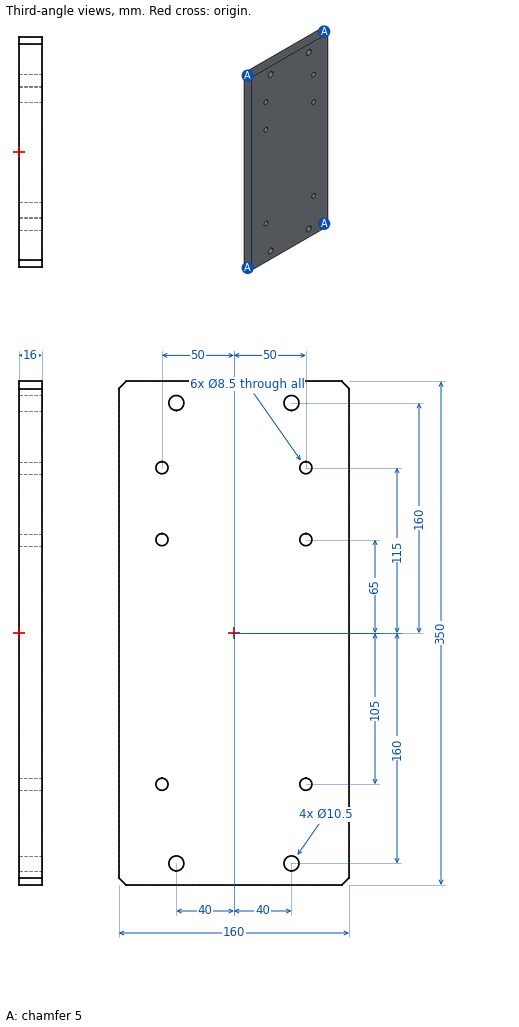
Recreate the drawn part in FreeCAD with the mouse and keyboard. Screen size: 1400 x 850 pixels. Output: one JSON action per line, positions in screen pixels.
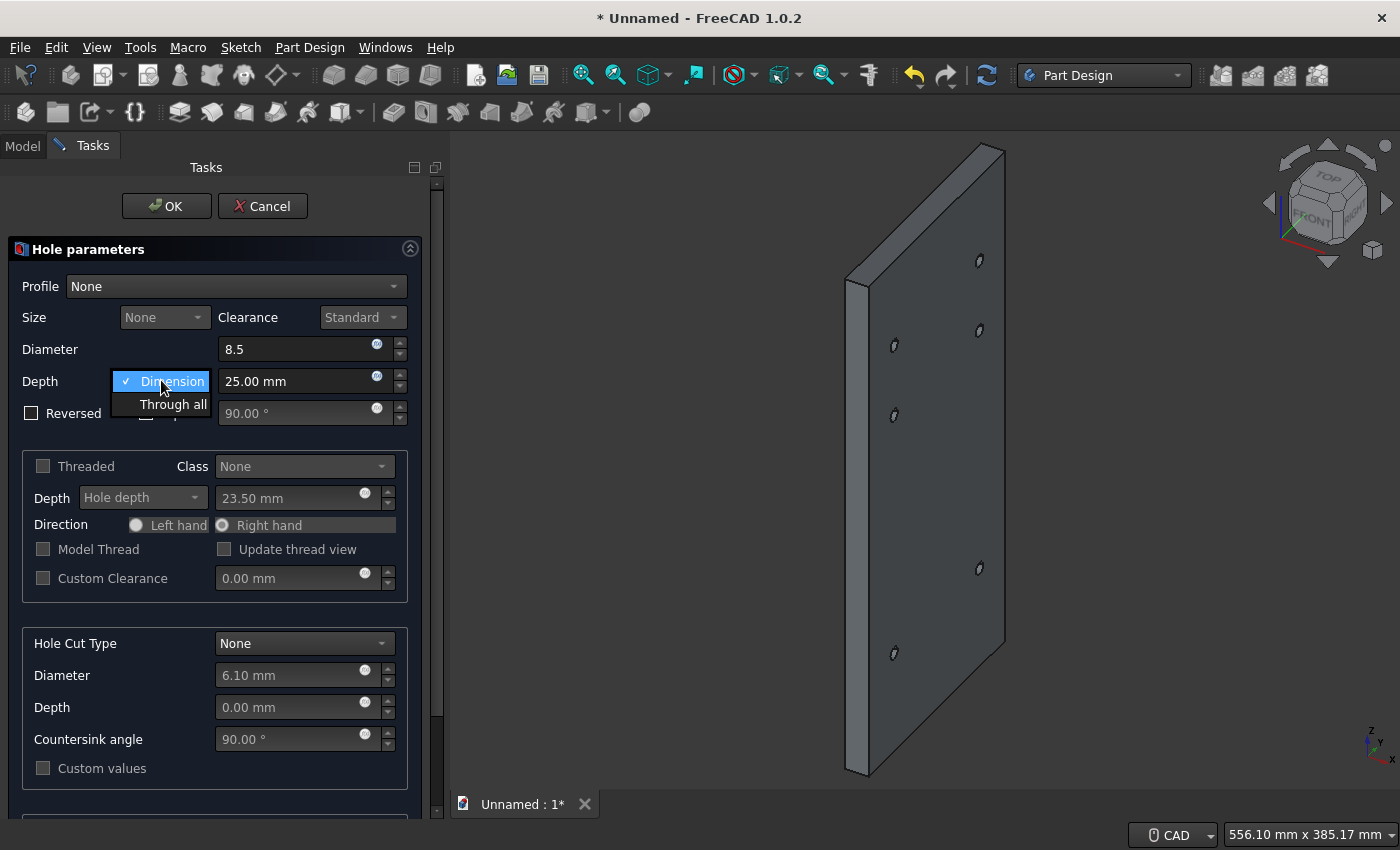
{"action": "left_click", "coordinate": [160, 404]}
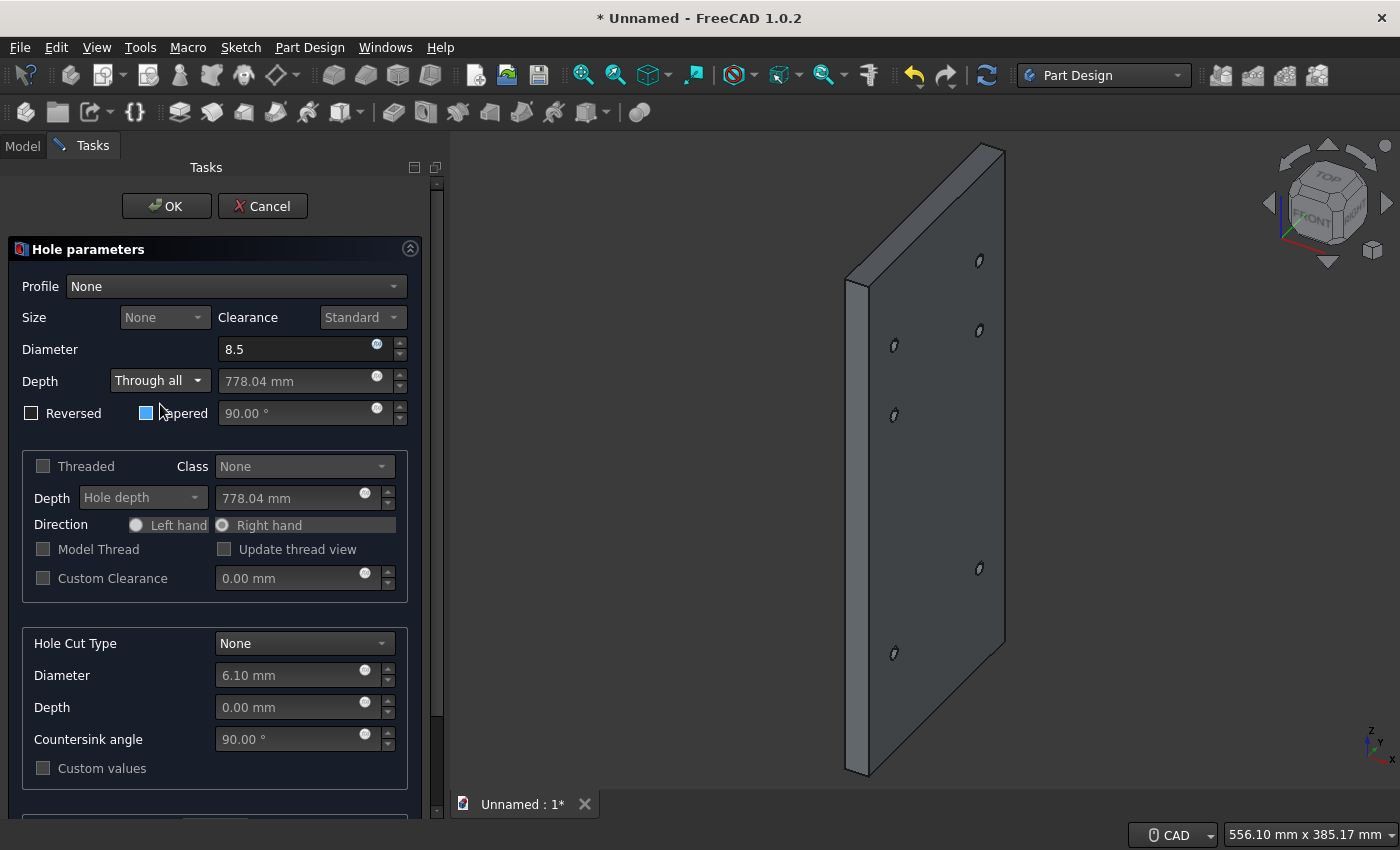
{"action": "left_click", "coordinate": [167, 206]}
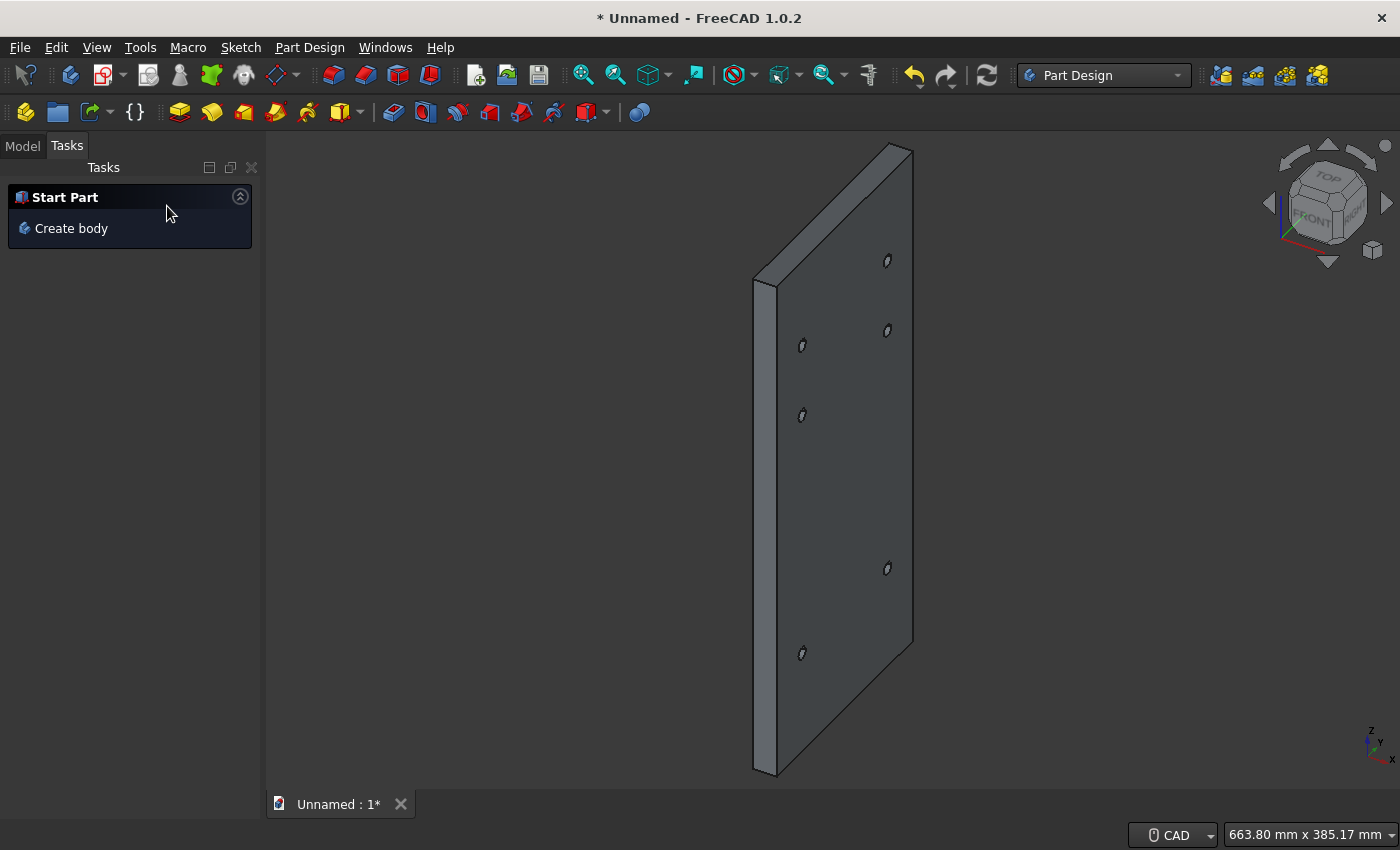
{"action": "key", "text": "6"}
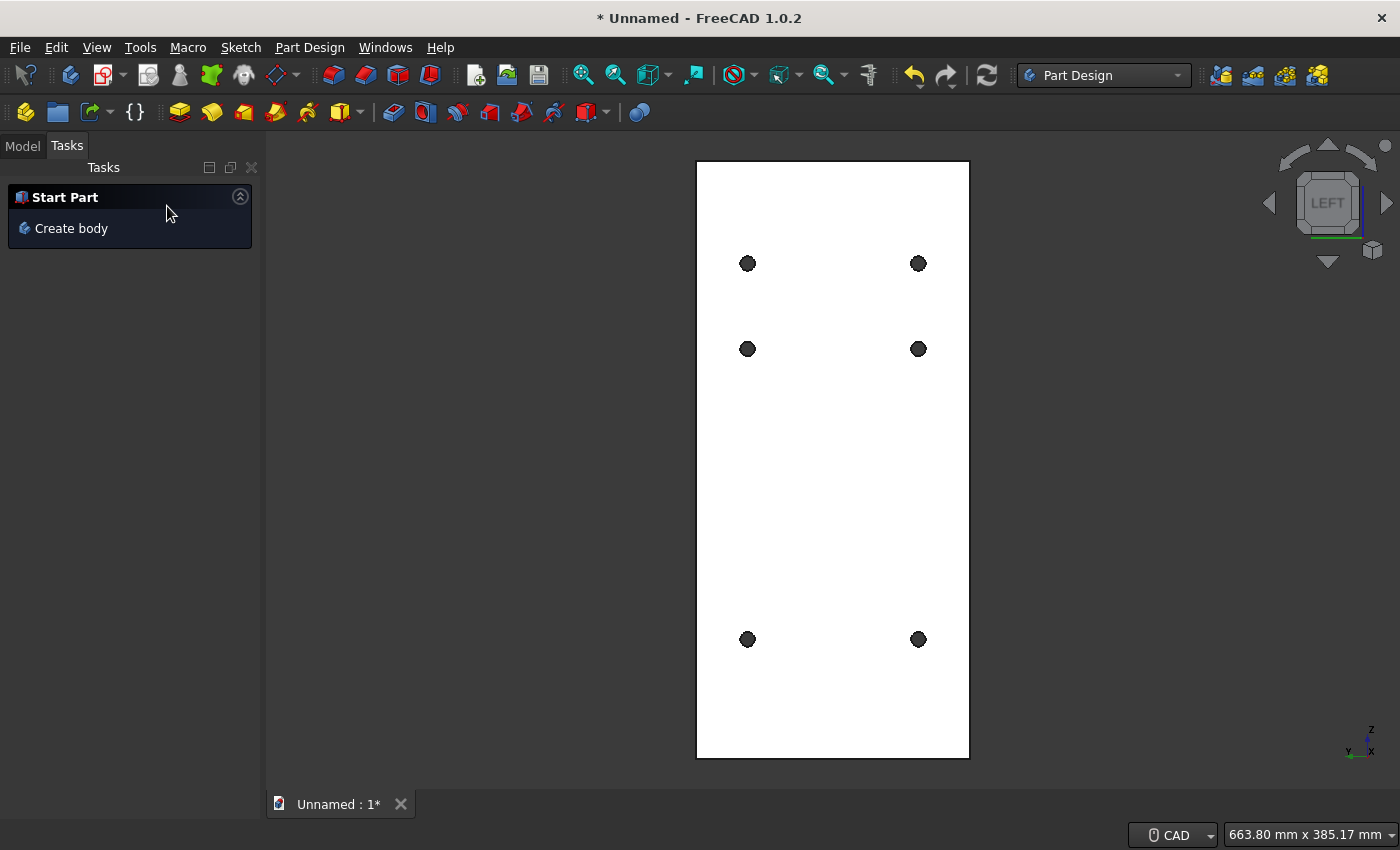
{"action": "left_click", "coordinate": [833, 459]}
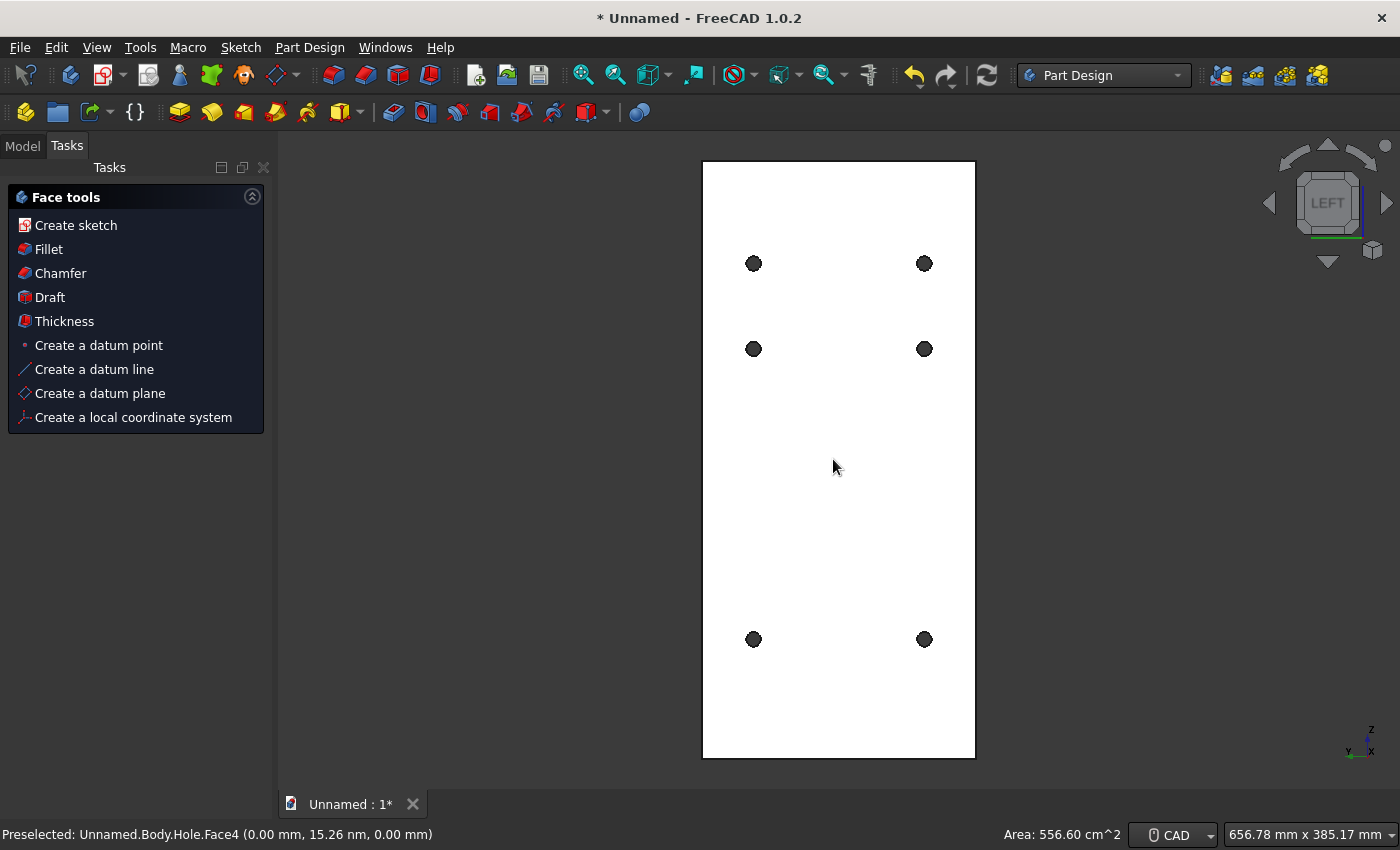
{"action": "left_click", "coordinate": [104, 76]}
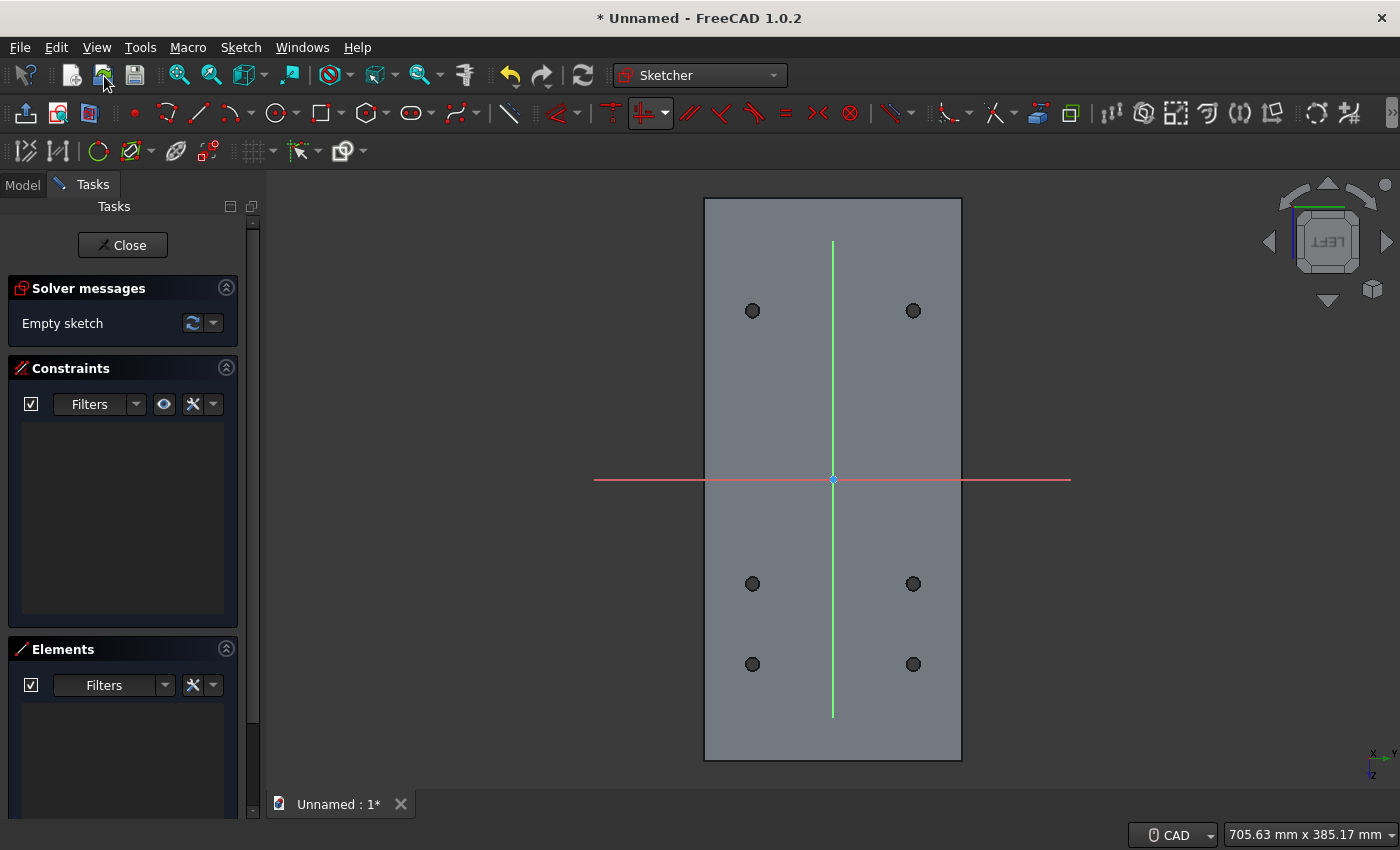
{"action": "scroll", "coordinate": [455, 480], "scroll_direction": "down", "scroll_amount": 1}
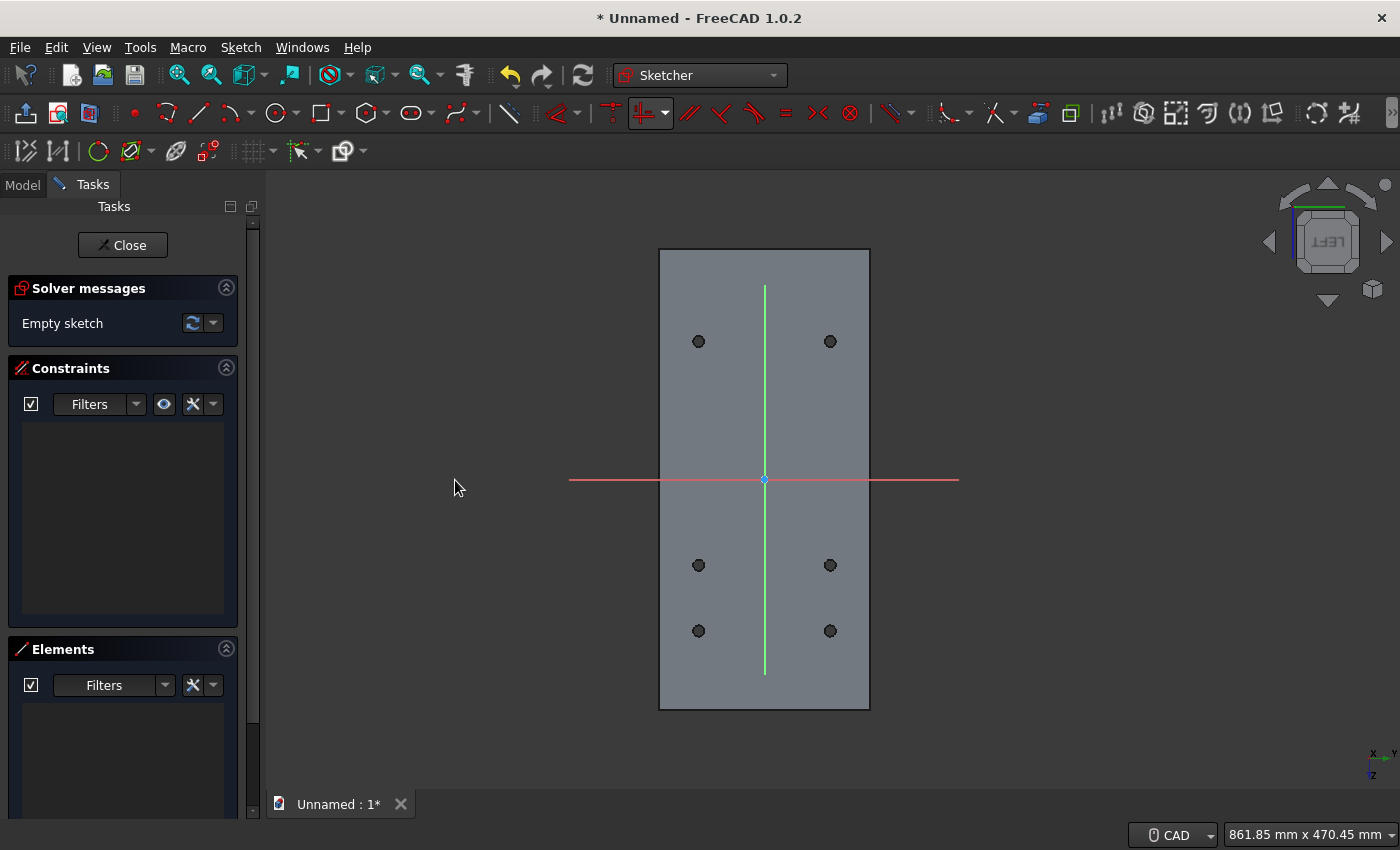
{"action": "left_click", "coordinate": [276, 114]}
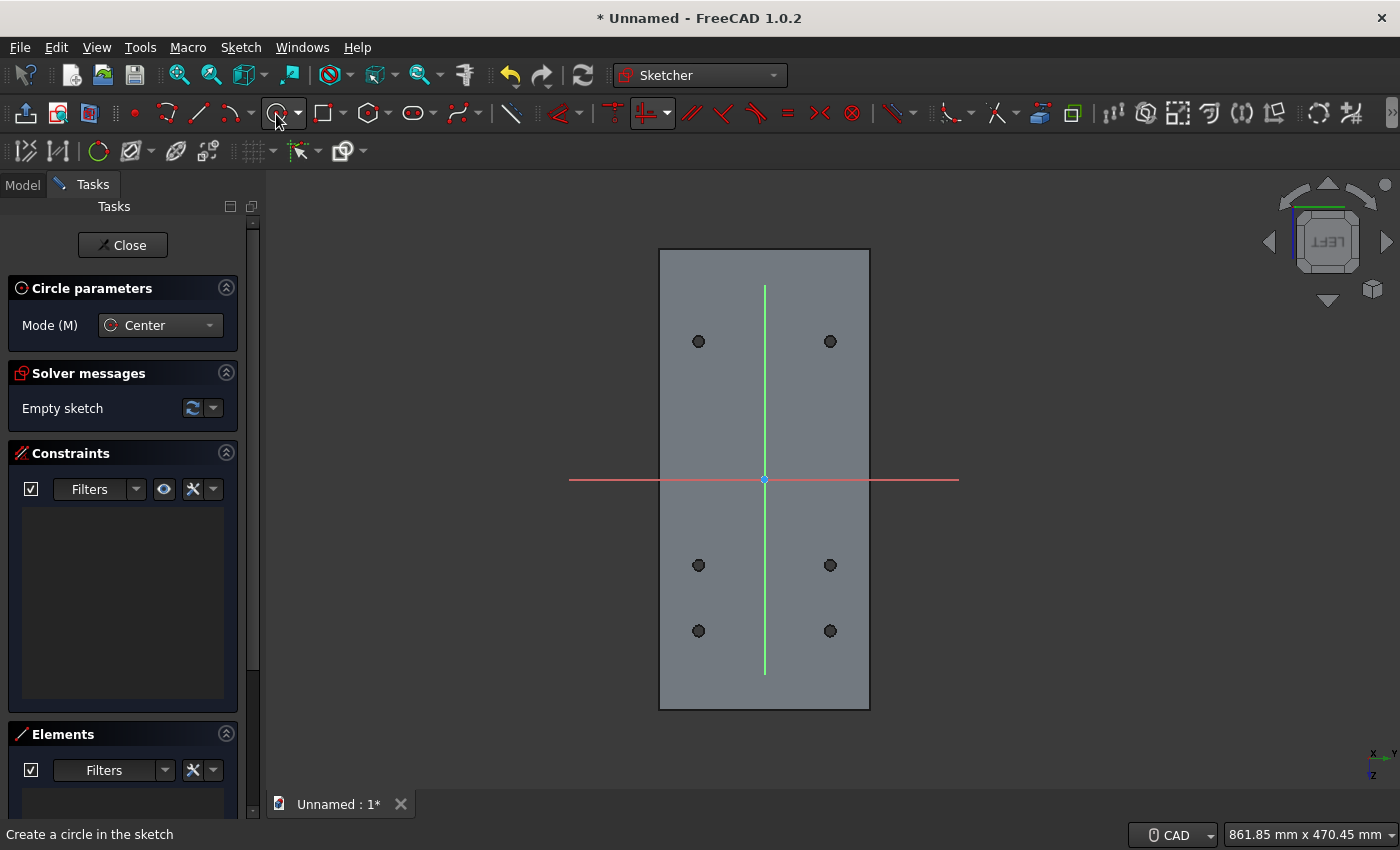
{"action": "scroll", "coordinate": [817, 269], "scroll_direction": "up", "scroll_amount": 6}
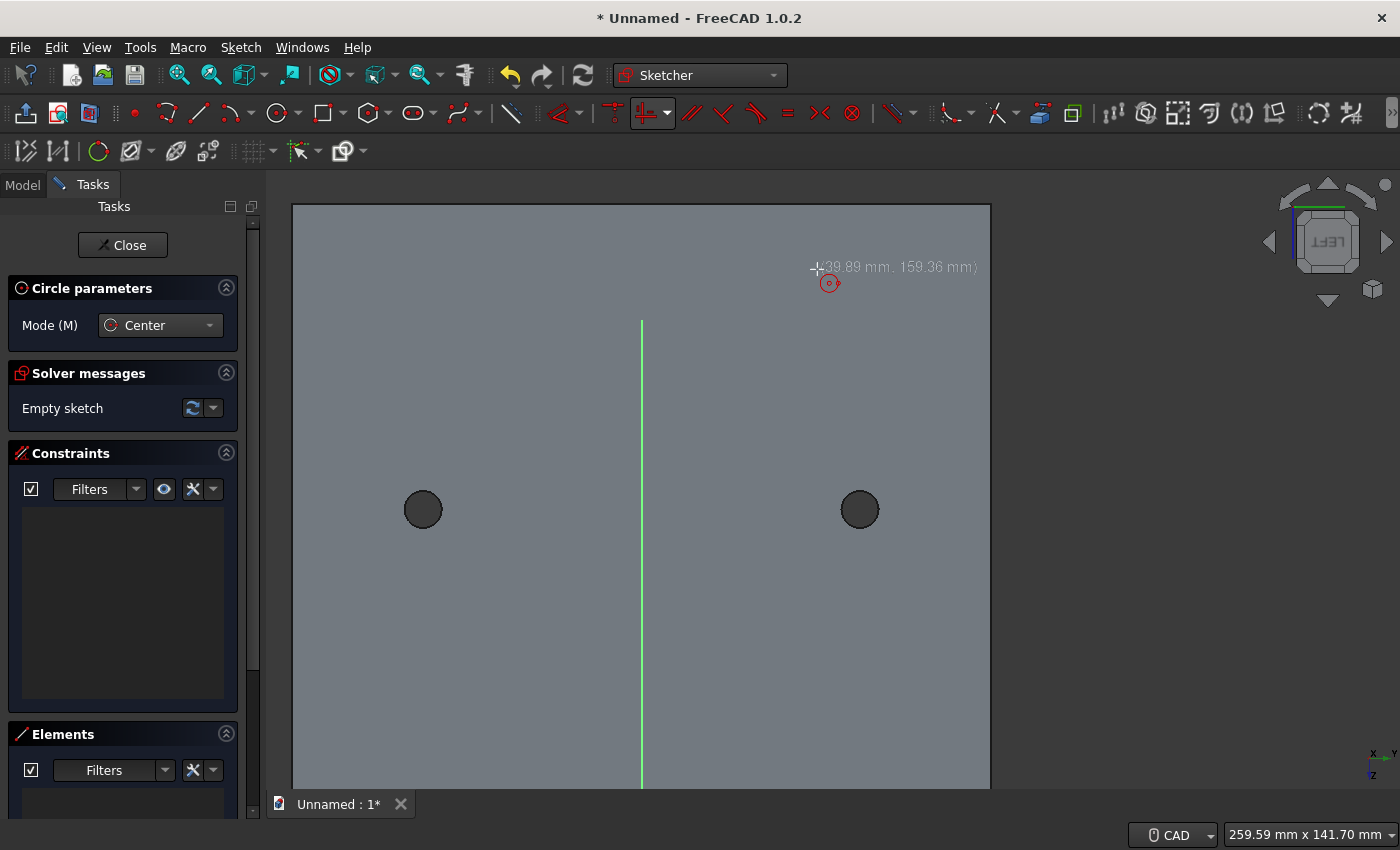
{"action": "left_click", "coordinate": [816, 269]}
{"action": "mouse_move", "coordinate": [833, 253]}